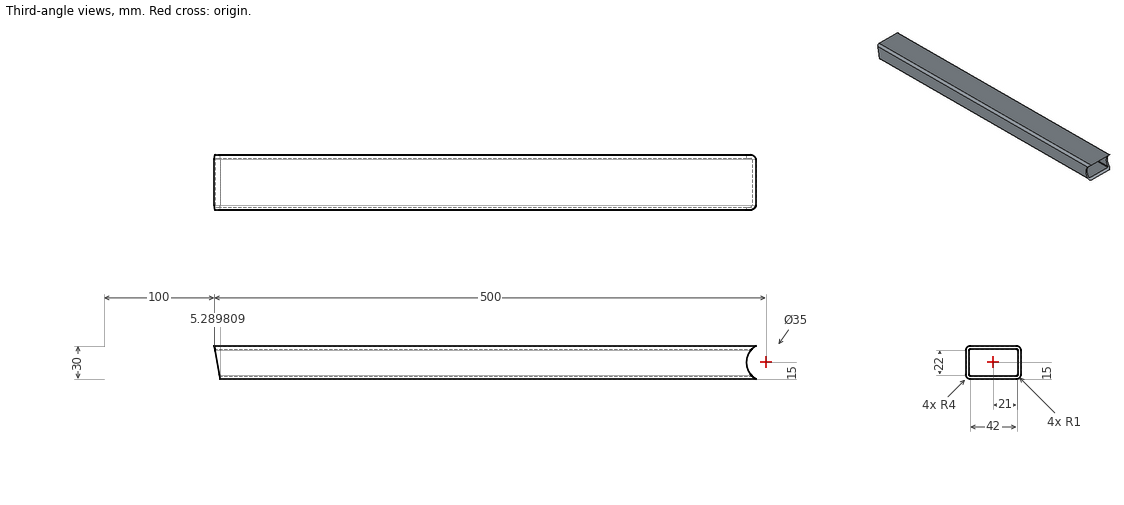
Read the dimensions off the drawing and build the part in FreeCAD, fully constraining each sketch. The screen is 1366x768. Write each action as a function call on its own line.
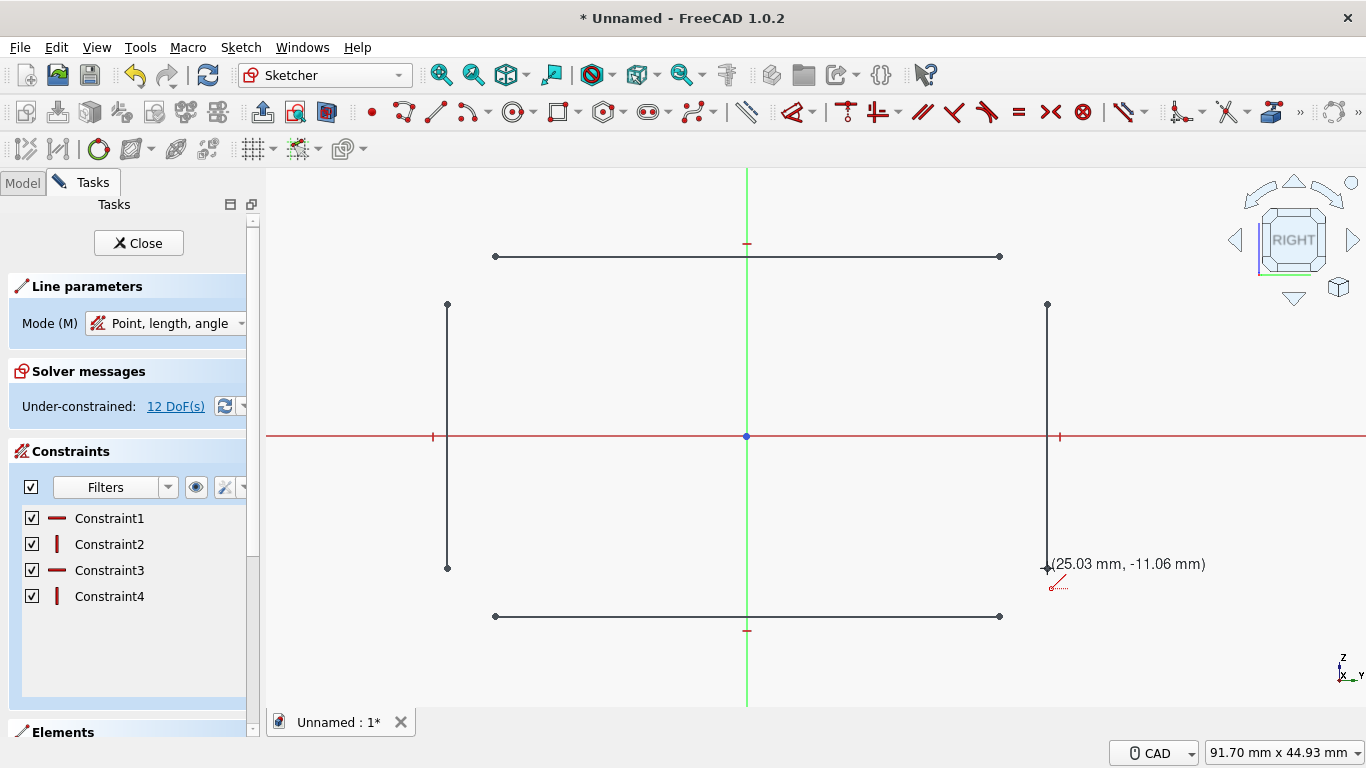
key(g)
key(3)
key(a)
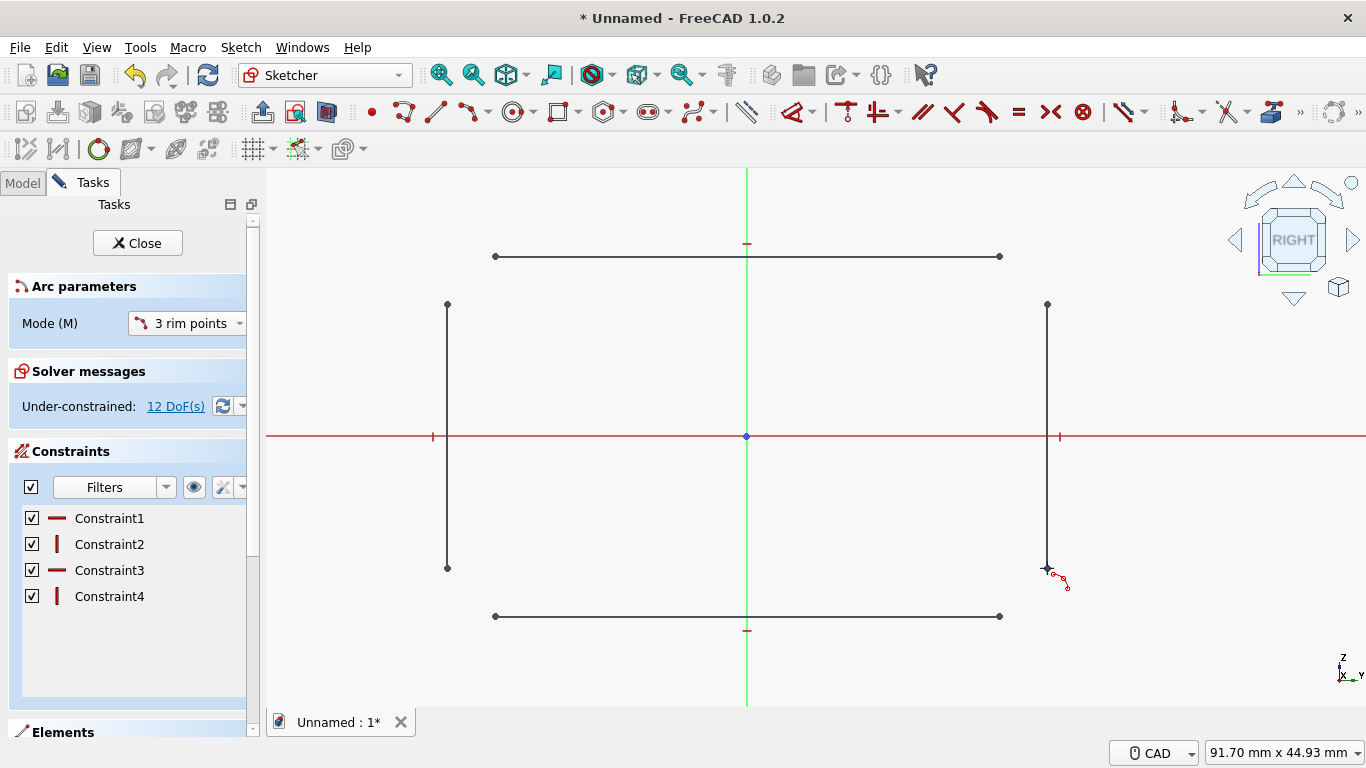
click(495, 617)
click(447, 569)
click(461, 602)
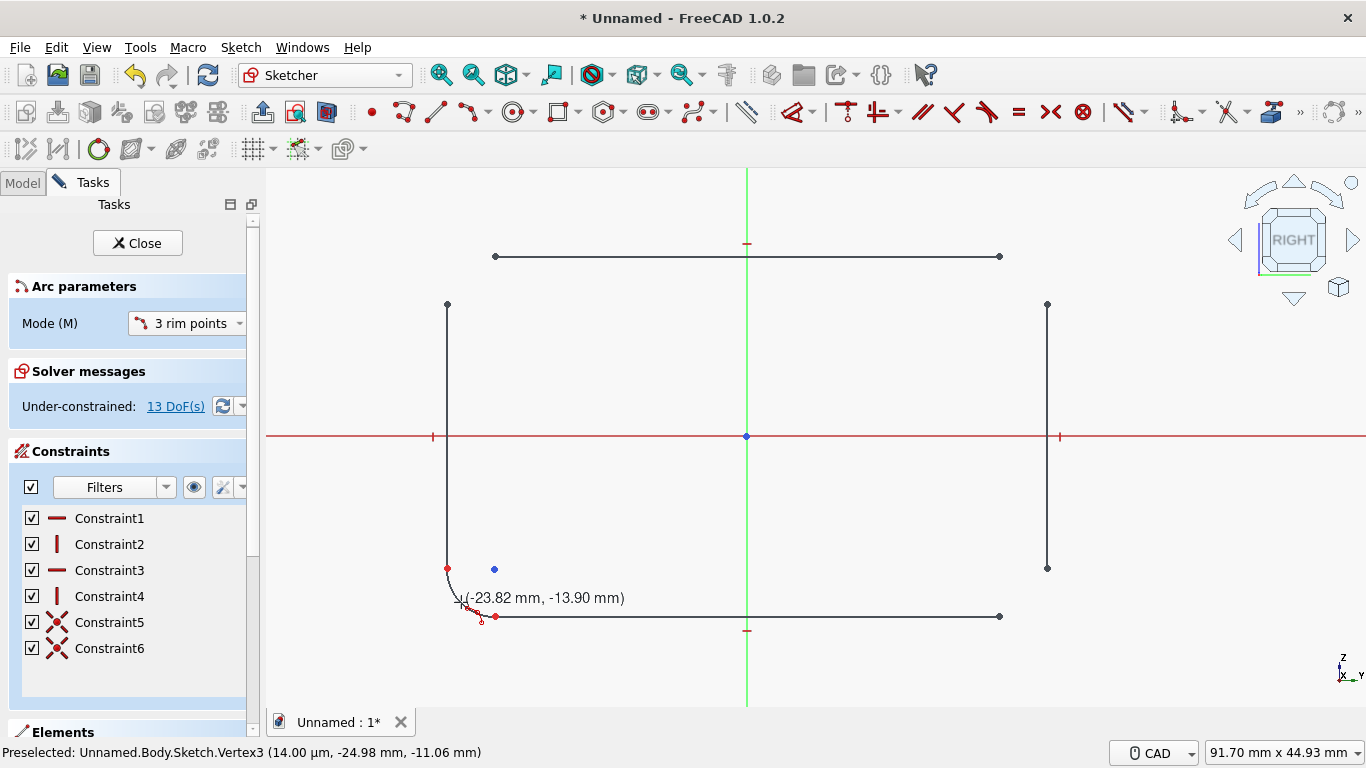
click(447, 305)
click(495, 257)
click(461, 270)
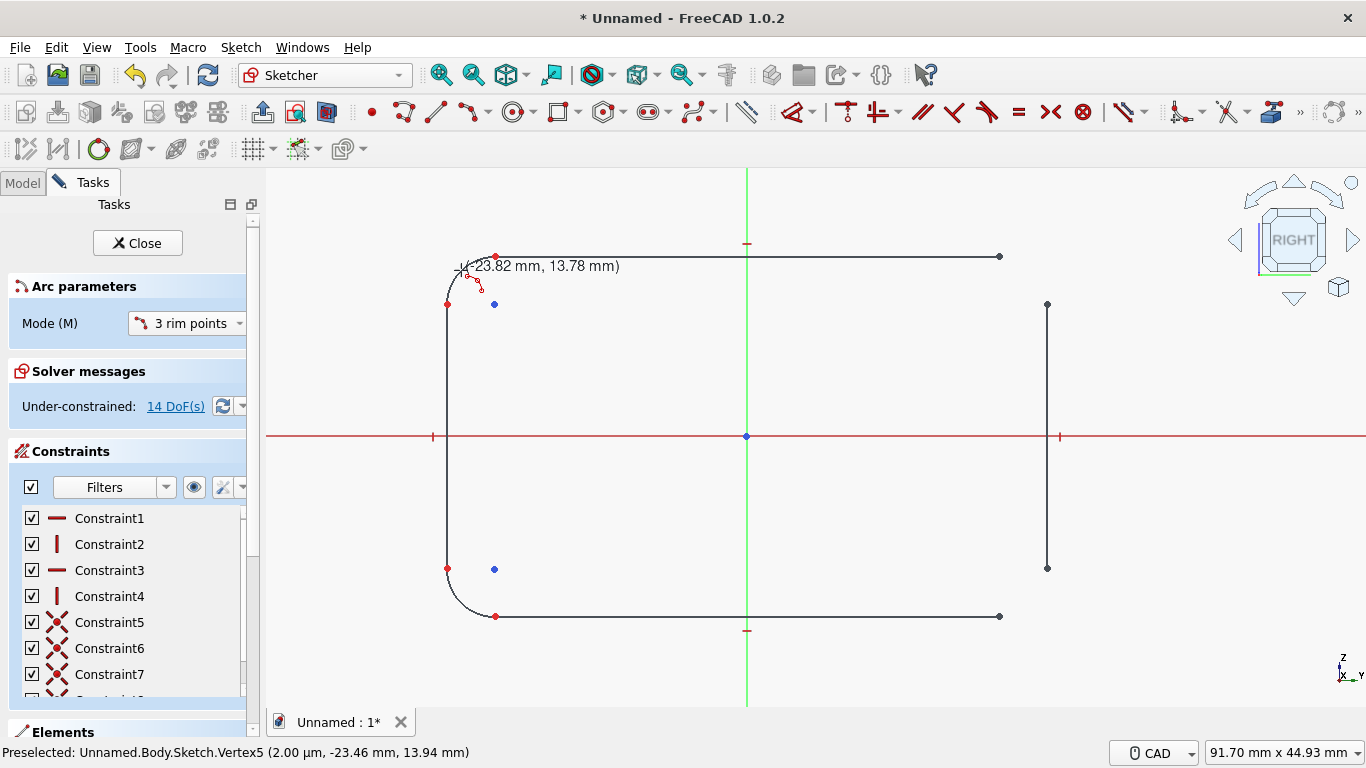
click(999, 257)
click(1047, 305)
click(1033, 270)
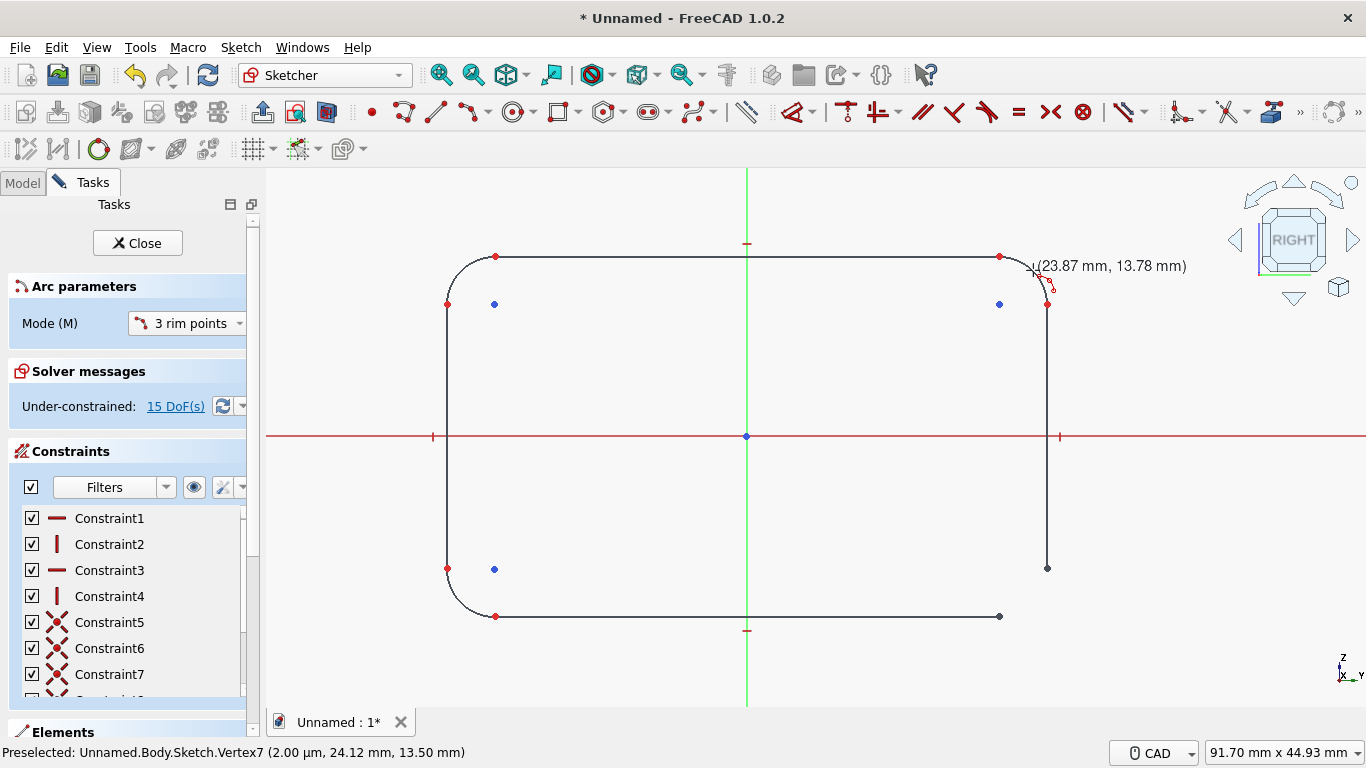
click(1047, 569)
click(999, 617)
click(1033, 602)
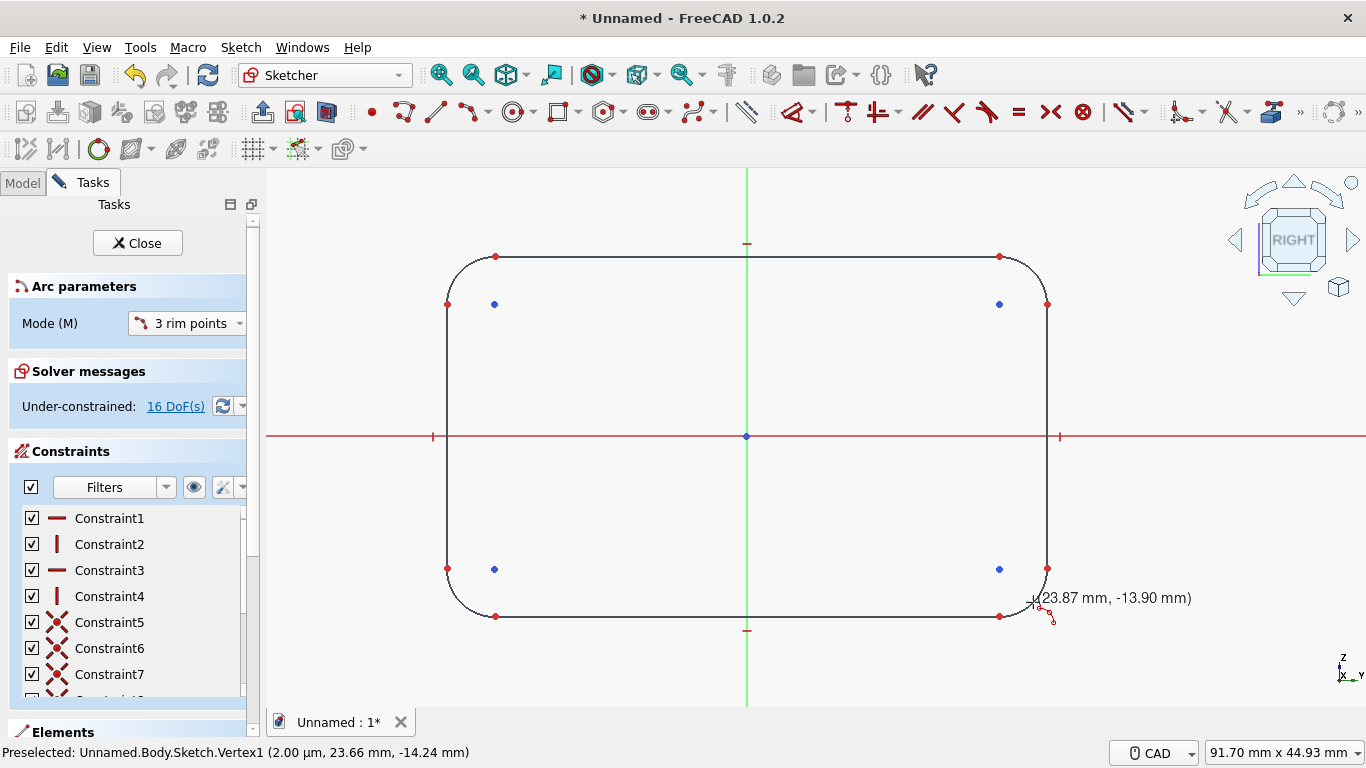
click(436, 112)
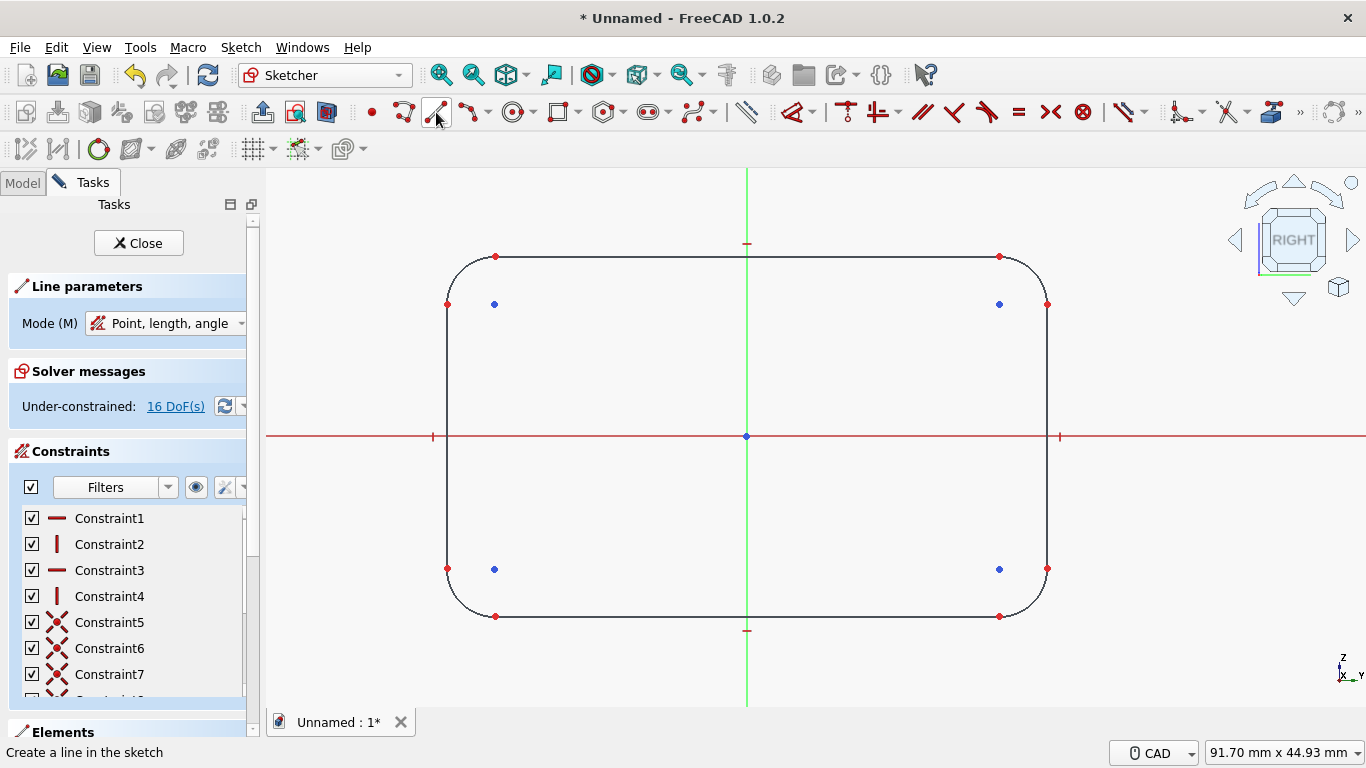
scroll(495, 580, up, 2)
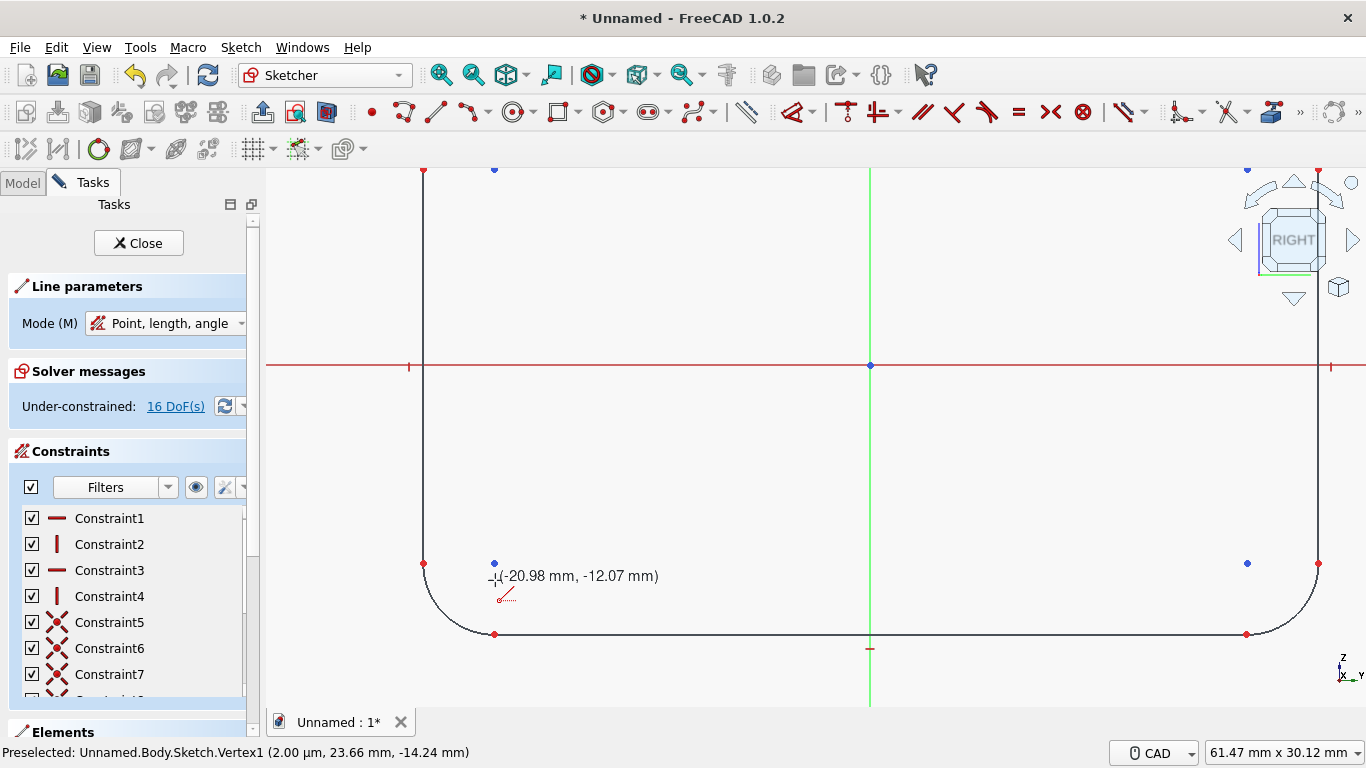
click(495, 580)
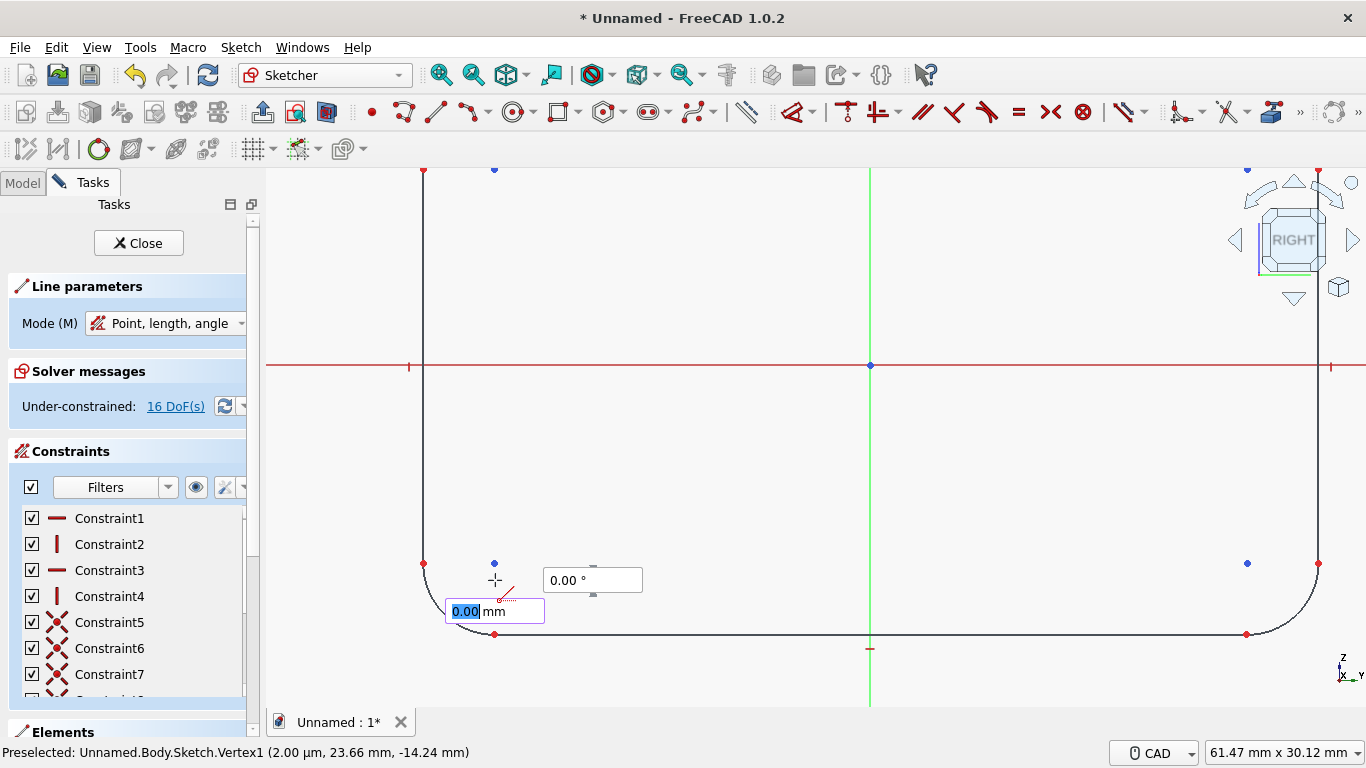
scroll(498, 584, down, 2)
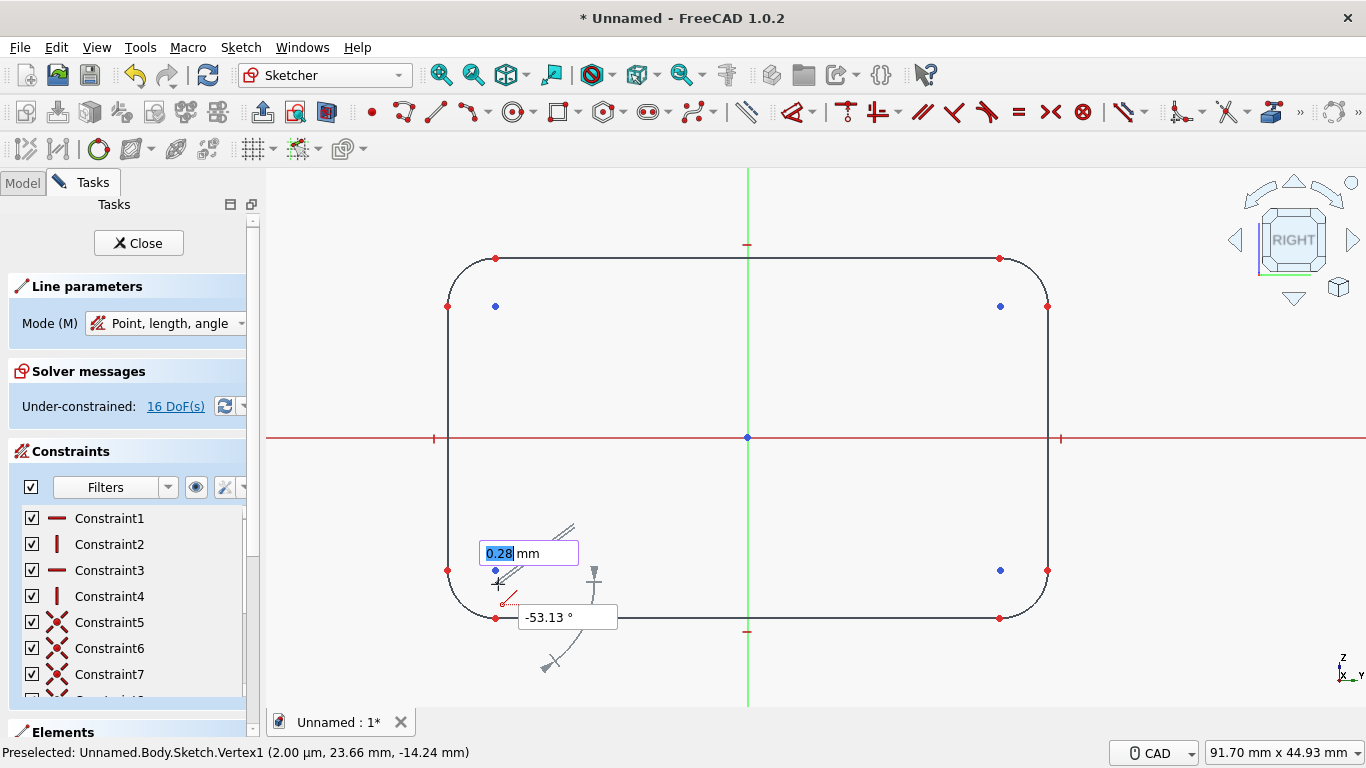
scroll(1000, 582, up, 2)